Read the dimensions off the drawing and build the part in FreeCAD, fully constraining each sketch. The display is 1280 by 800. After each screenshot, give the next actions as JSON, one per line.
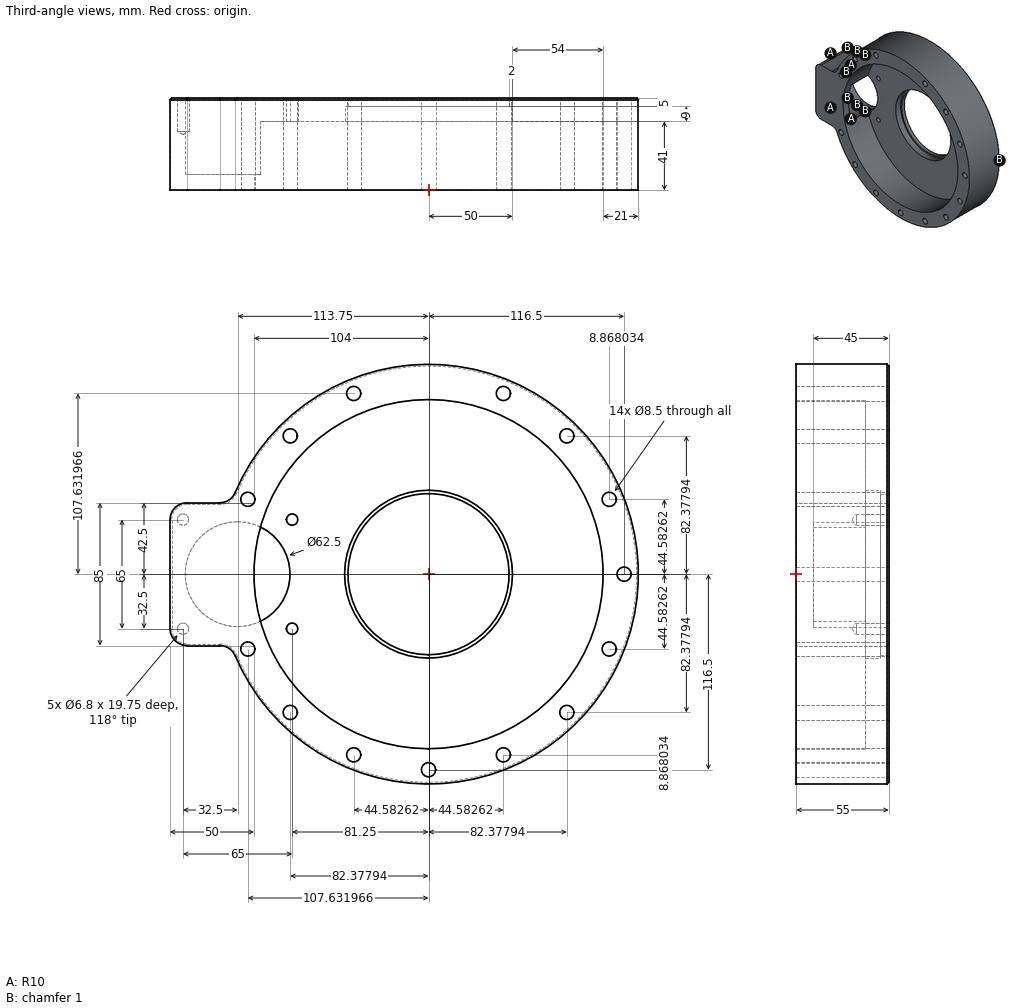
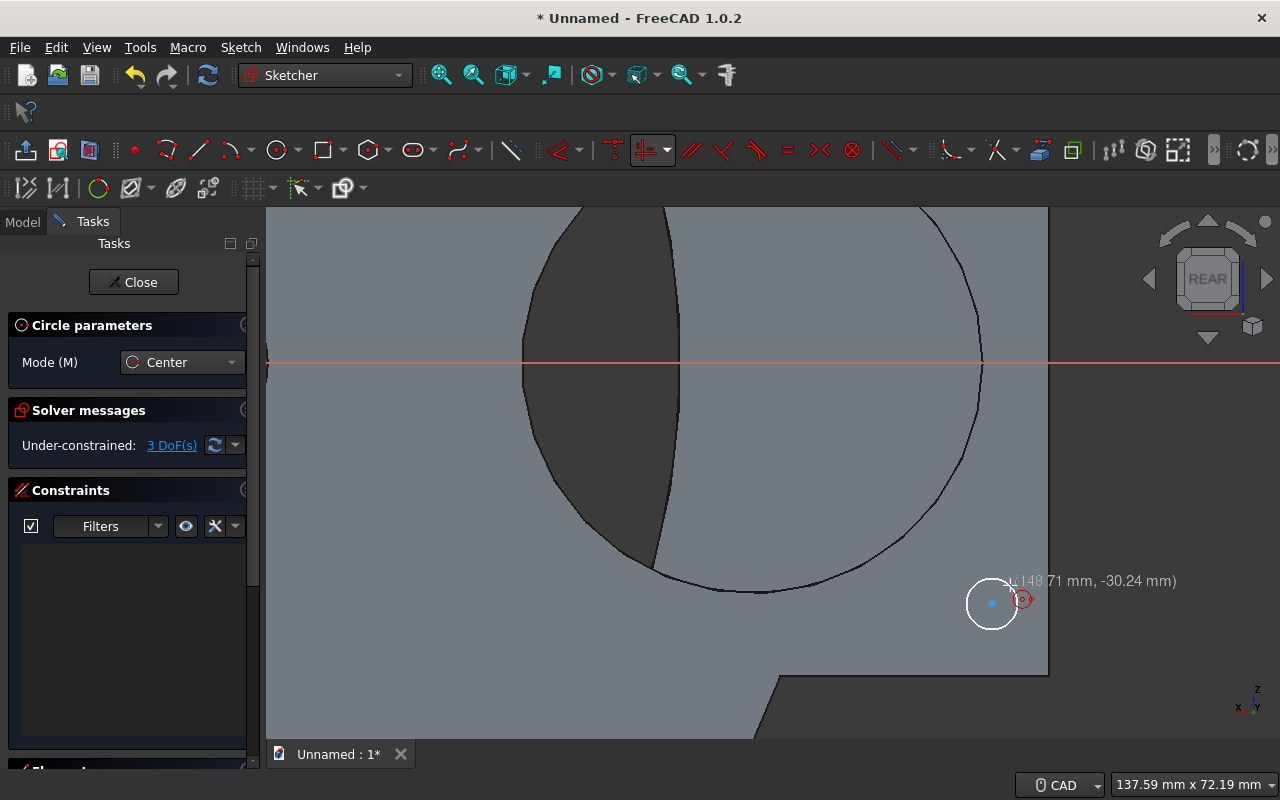
{"action": "left_click", "coordinate": [752, 363]}
{"action": "left_click", "coordinate": [770, 345]}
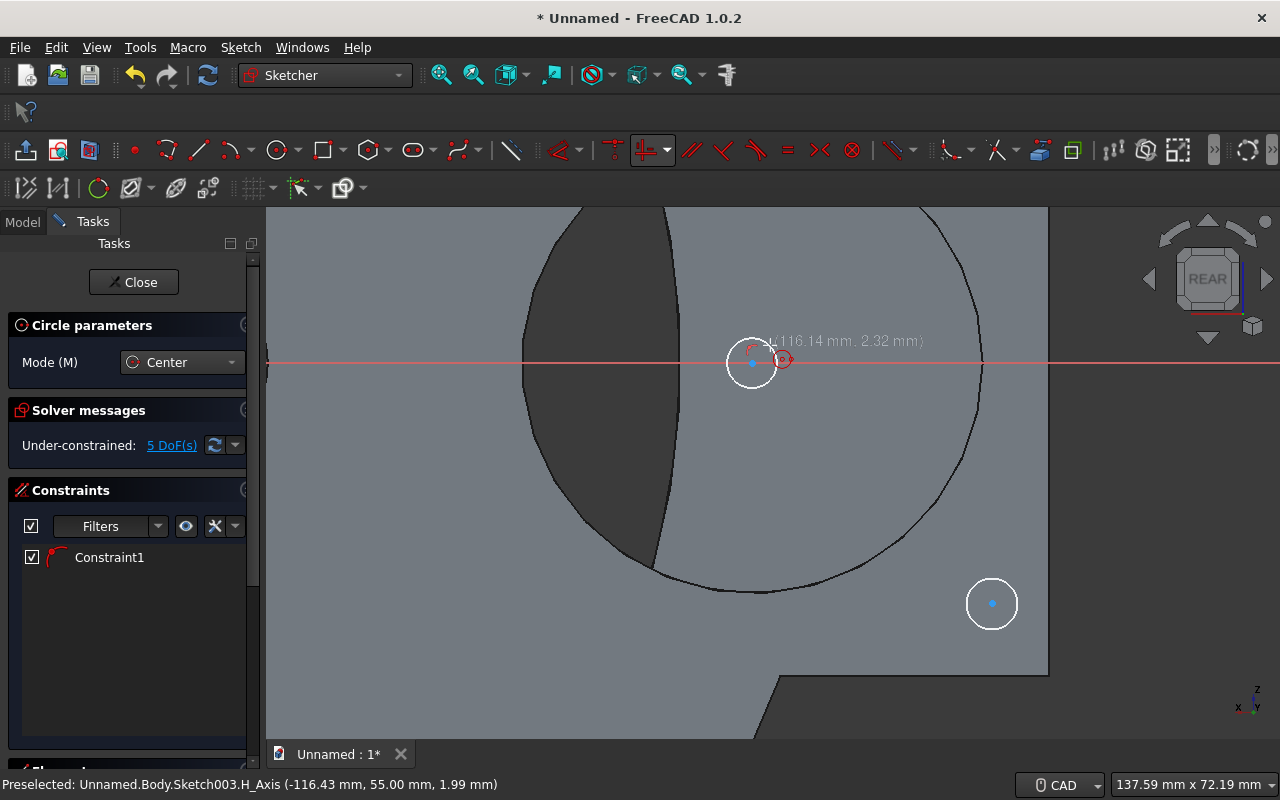
{"action": "left_click", "coordinate": [513, 603]}
{"action": "left_click", "coordinate": [531, 585]}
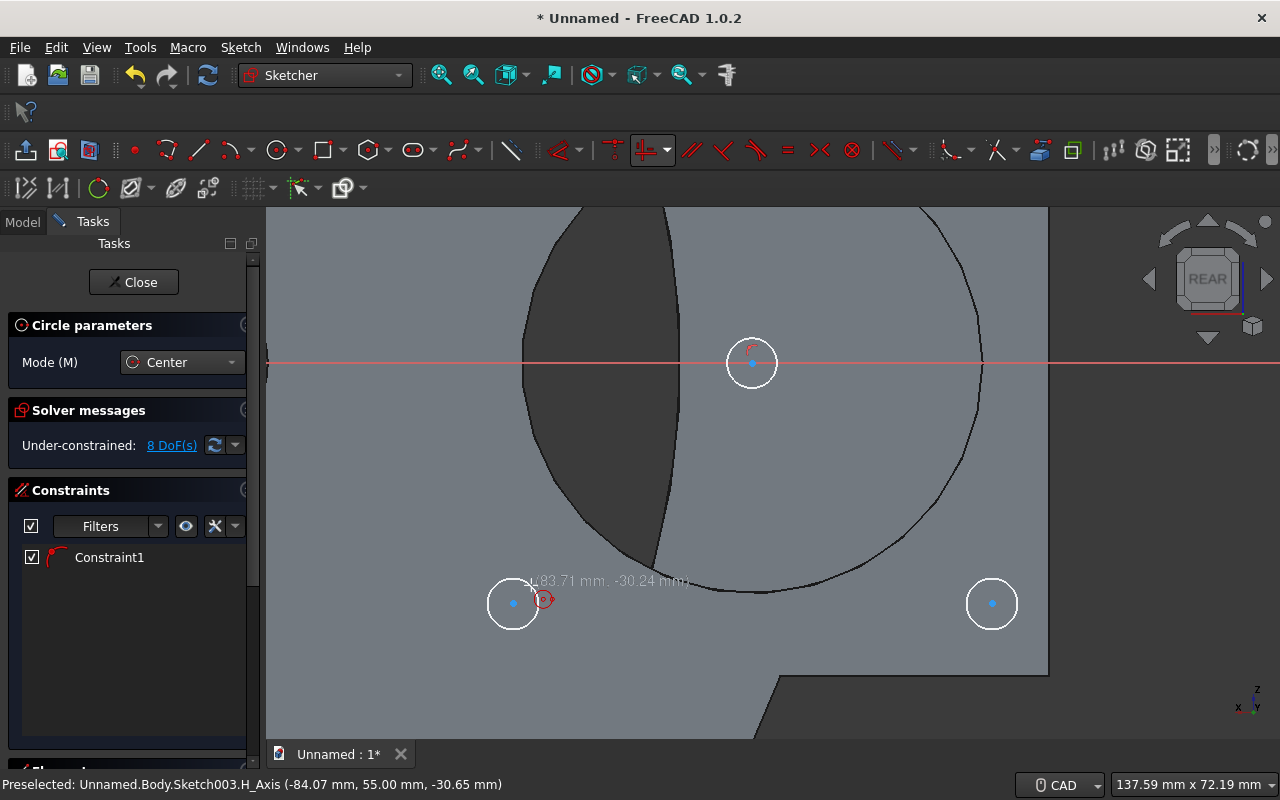
{"action": "scroll", "coordinate": [995, 607], "scroll_direction": "down", "scroll_amount": 3}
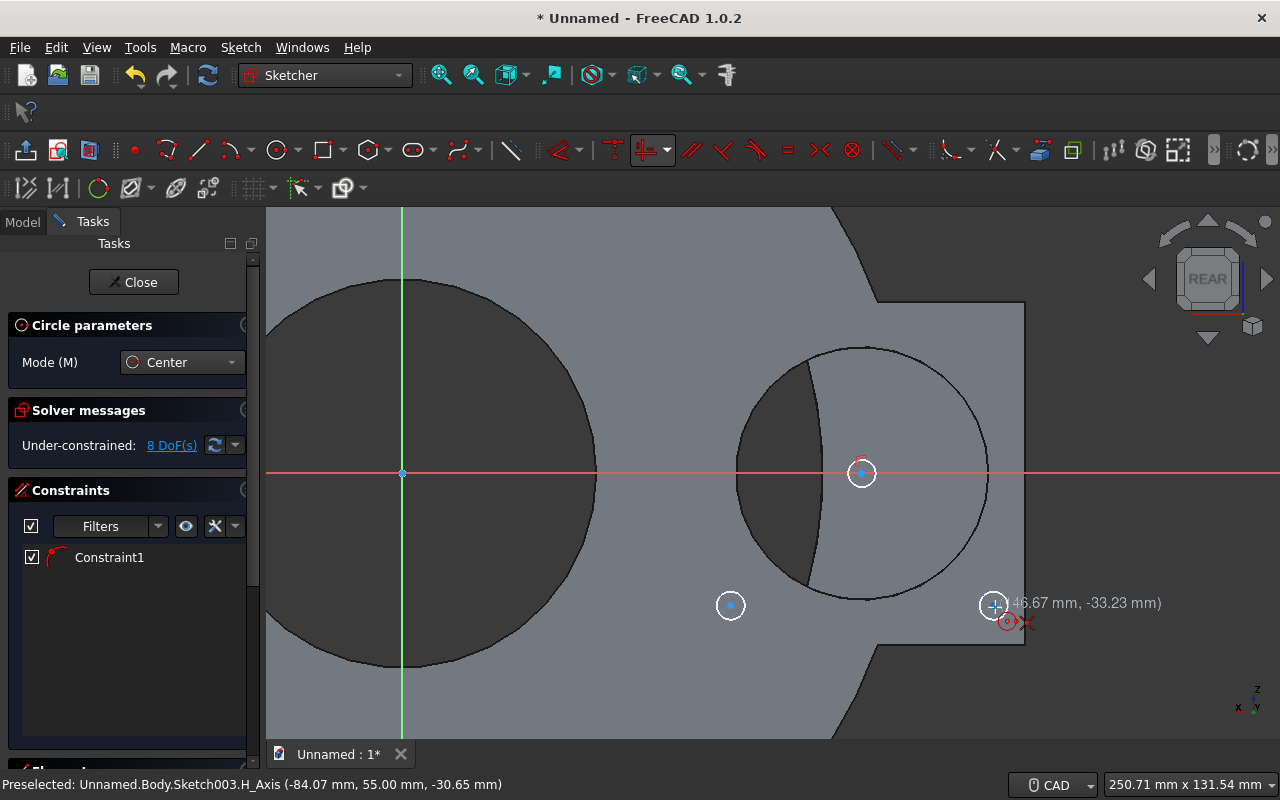
{"action": "scroll", "coordinate": [994, 342], "scroll_direction": "up", "scroll_amount": 3}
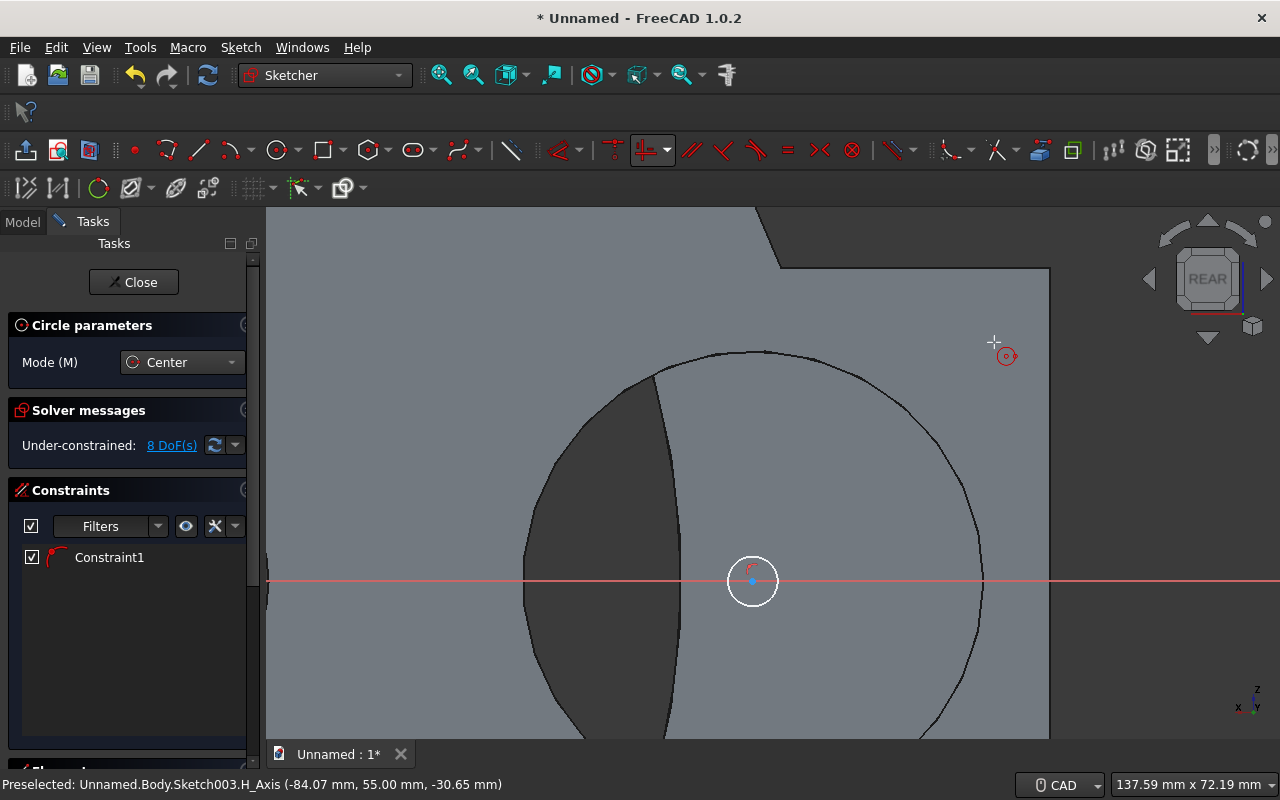
{"action": "left_click", "coordinate": [993, 342]}
{"action": "left_click", "coordinate": [1010, 324]}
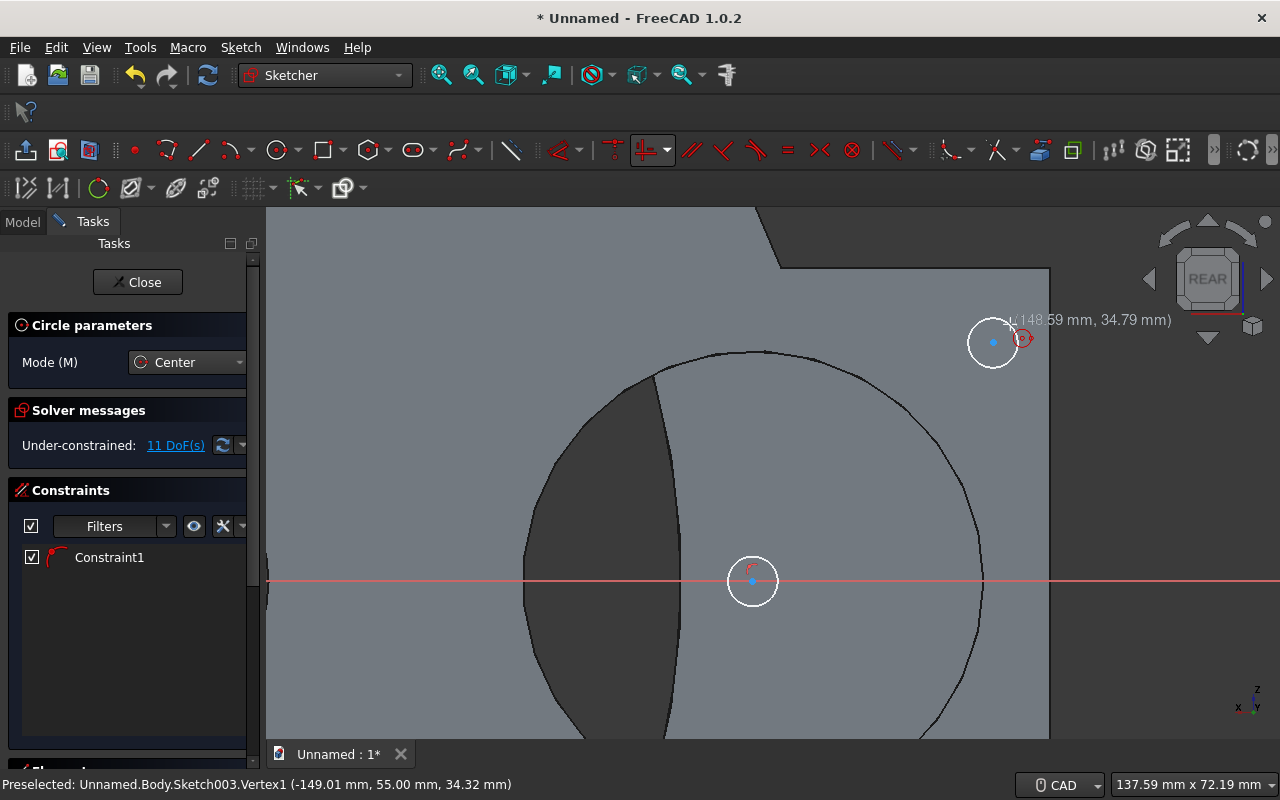
{"action": "left_click", "coordinate": [514, 342]}
{"action": "left_click", "coordinate": [531, 324]}
{"action": "key", "text": "Escape"}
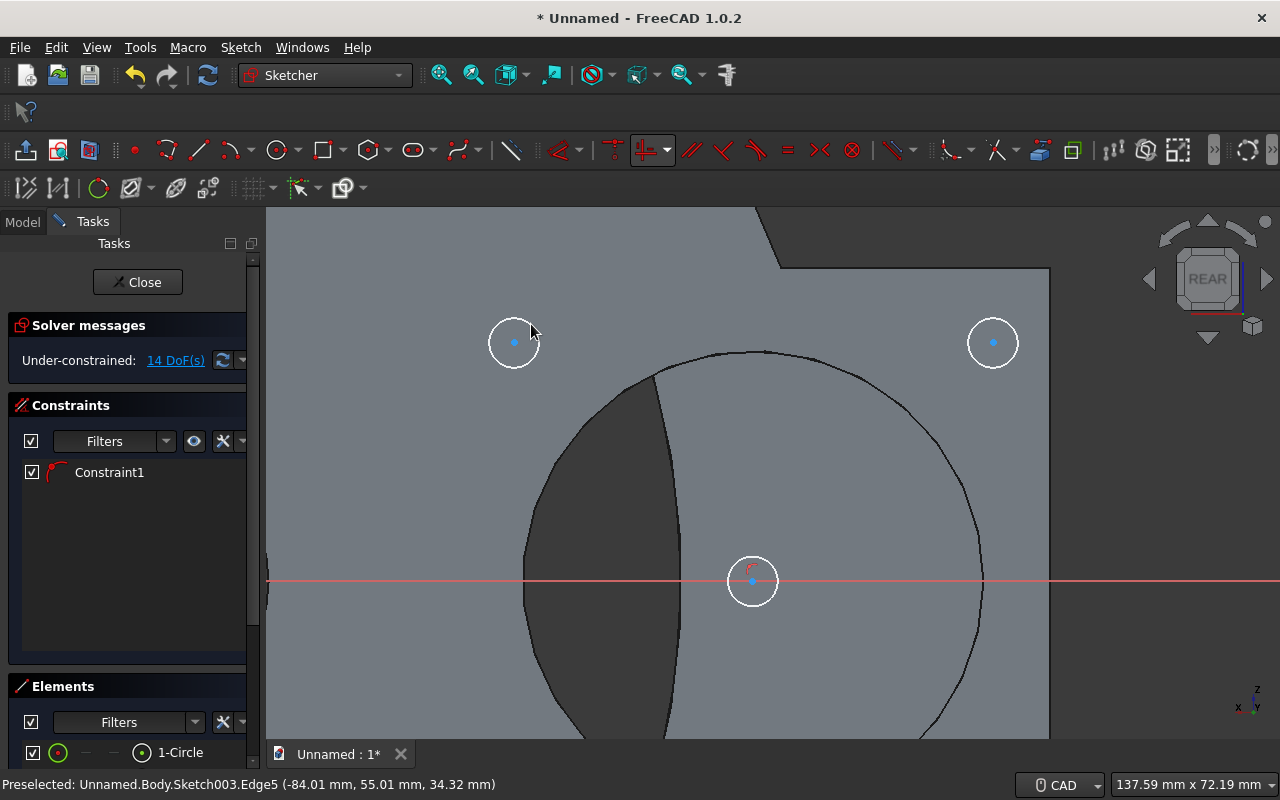
{"action": "scroll", "coordinate": [994, 341], "scroll_direction": "down", "scroll_amount": 3}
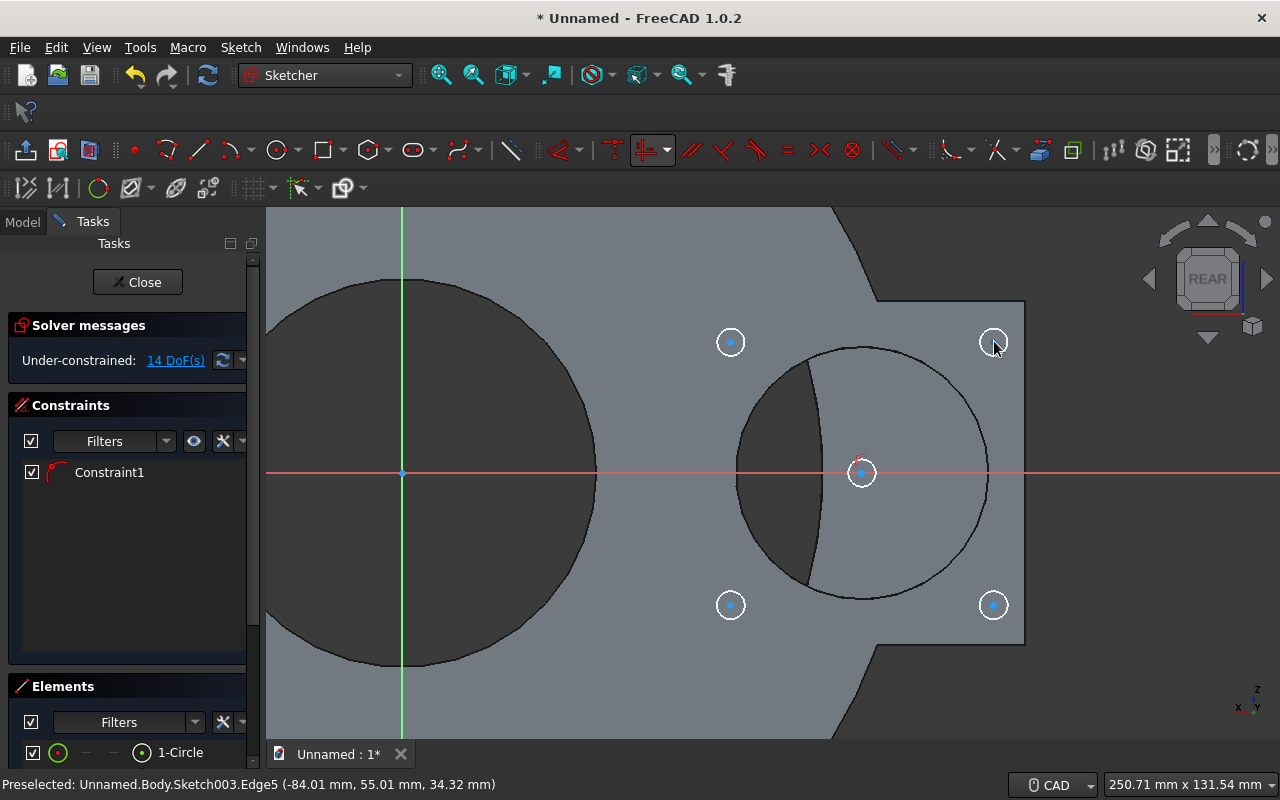
{"action": "left_click", "coordinate": [1004, 595]}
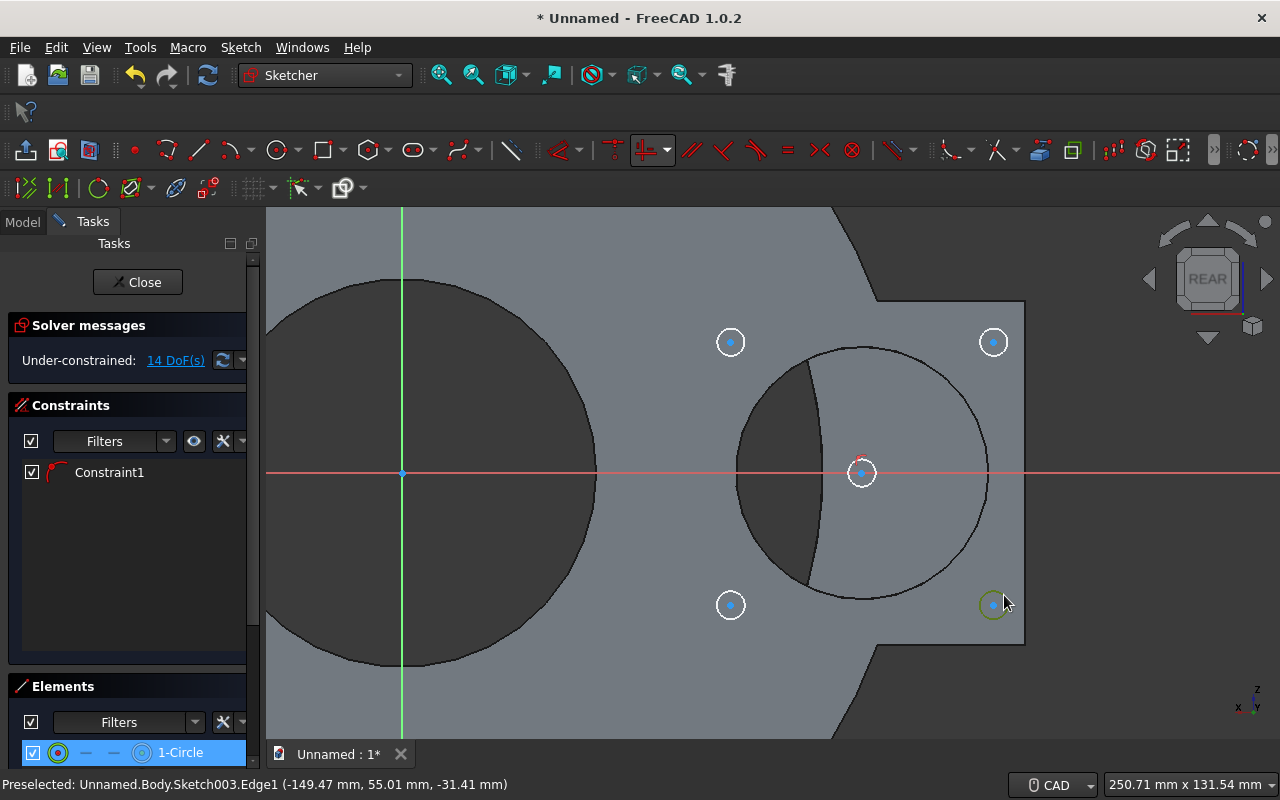
{"action": "scroll", "coordinate": [872, 463], "scroll_direction": "up", "scroll_amount": 2}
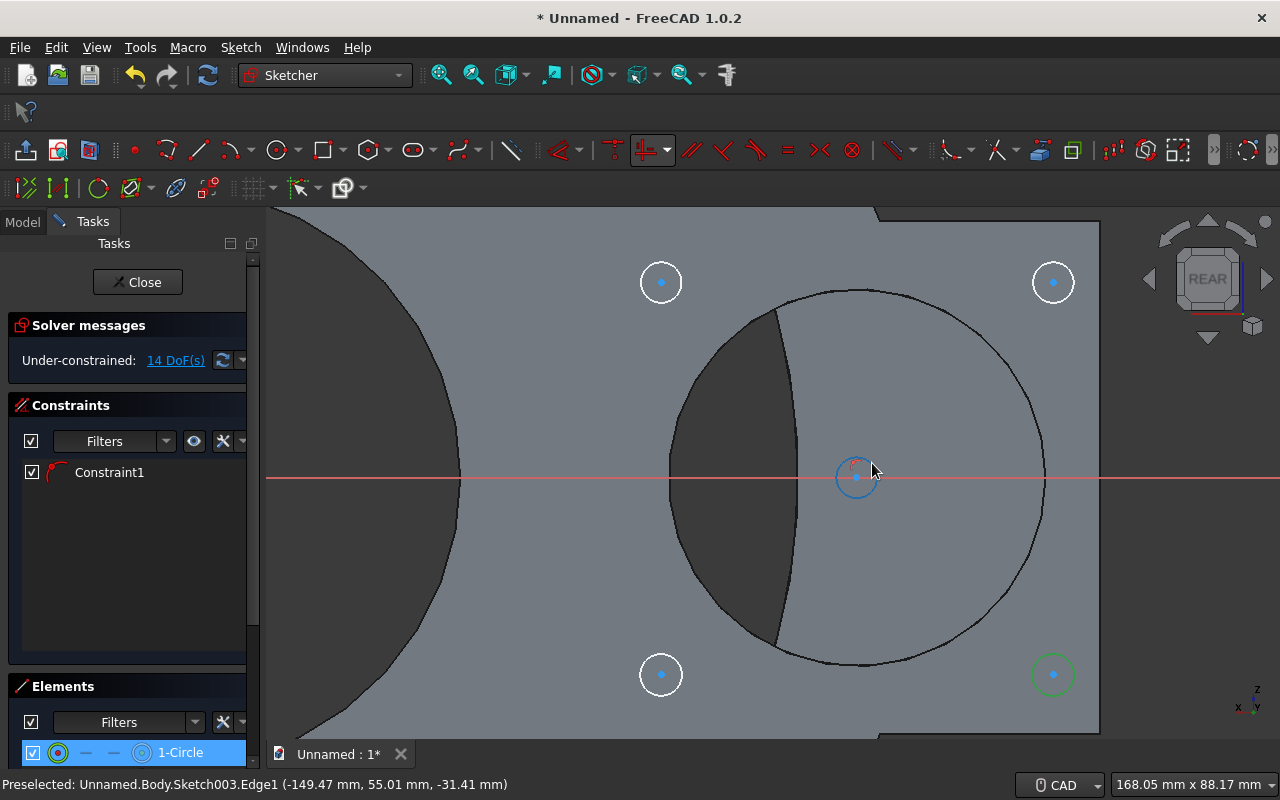
{"action": "left_click", "coordinate": [871, 463]}